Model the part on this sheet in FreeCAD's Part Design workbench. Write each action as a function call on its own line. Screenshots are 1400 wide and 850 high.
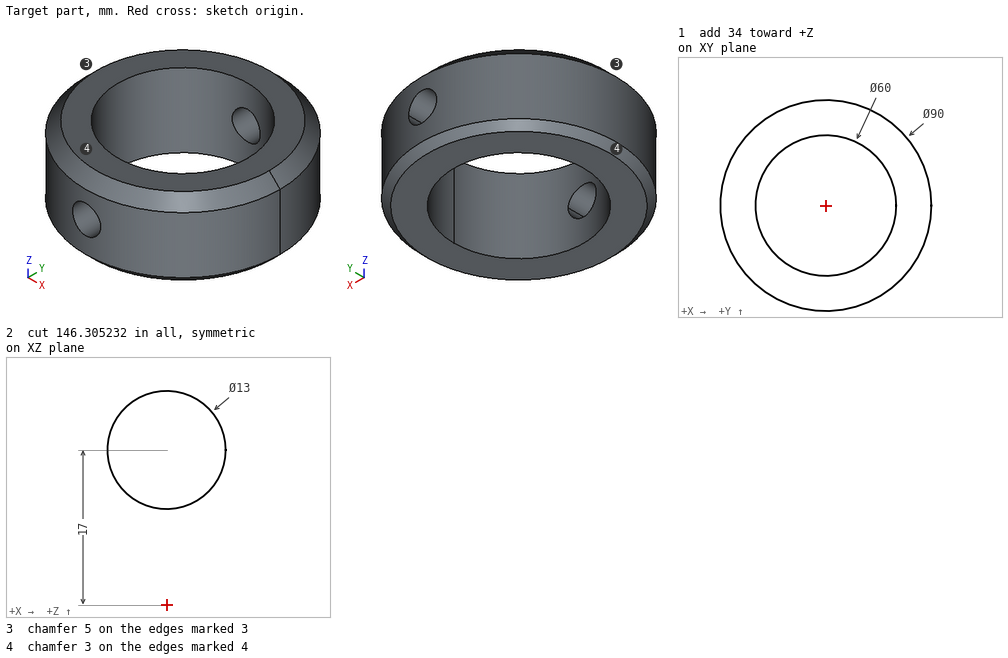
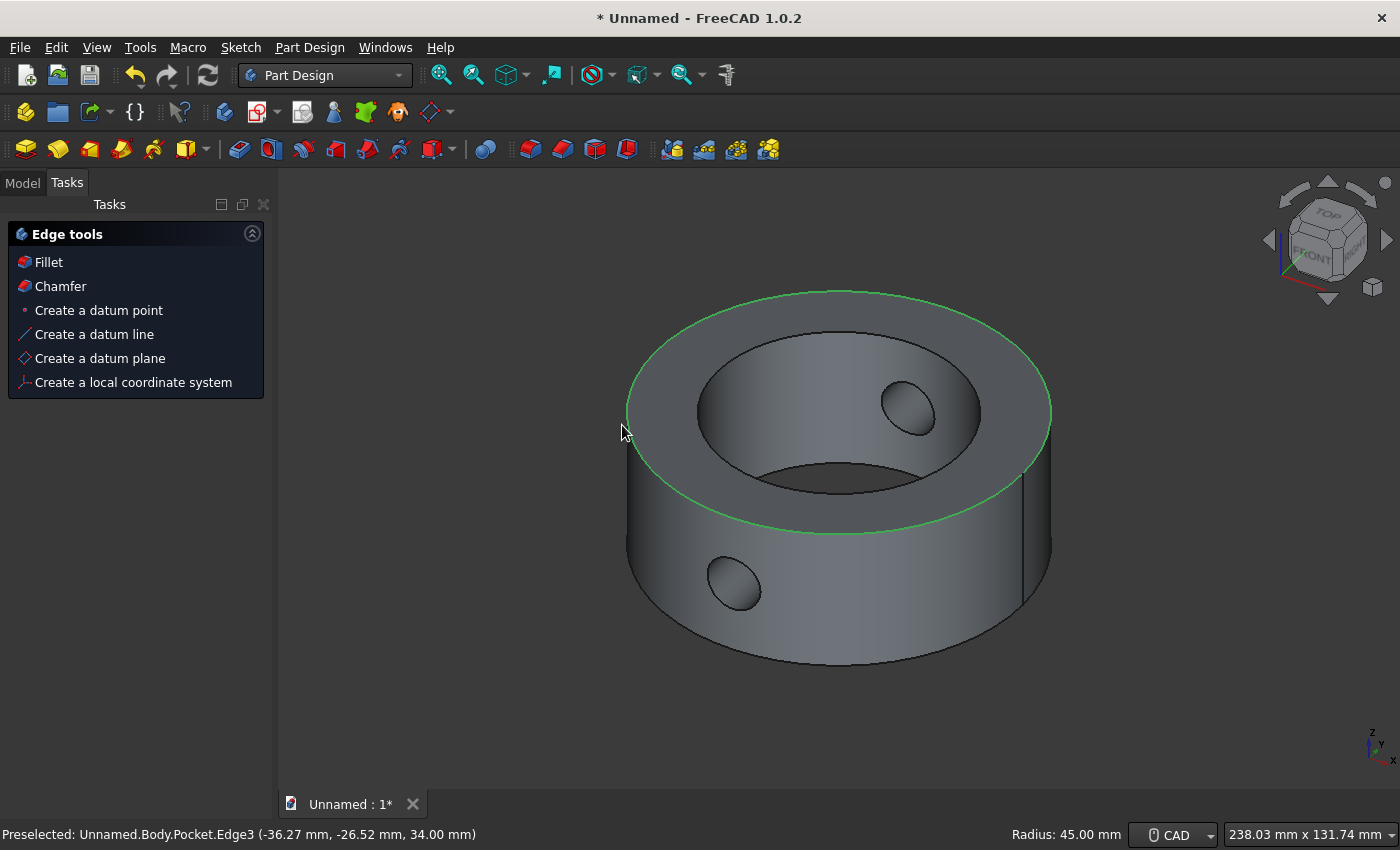
click(564, 150)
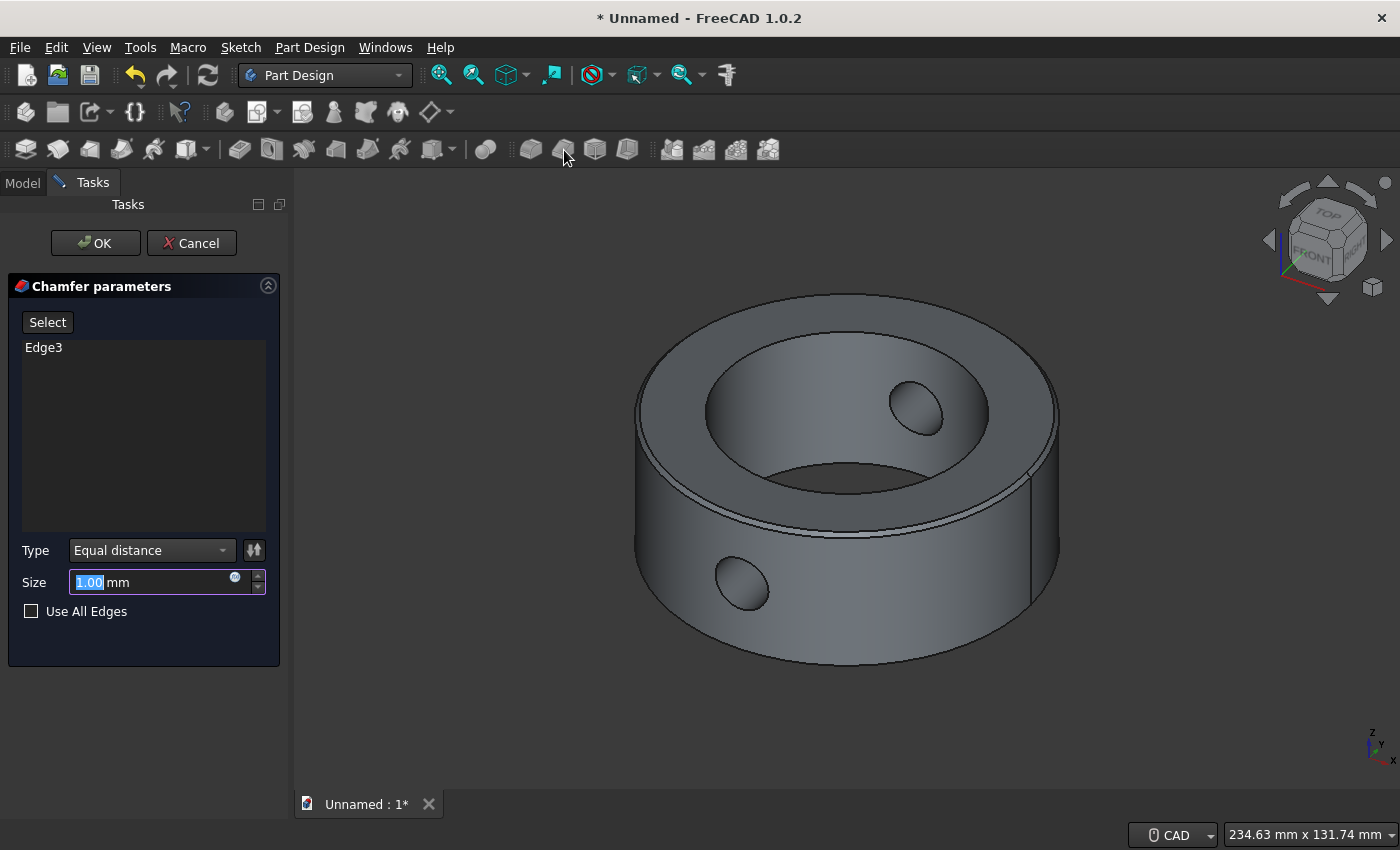
text(5)
key(Tab)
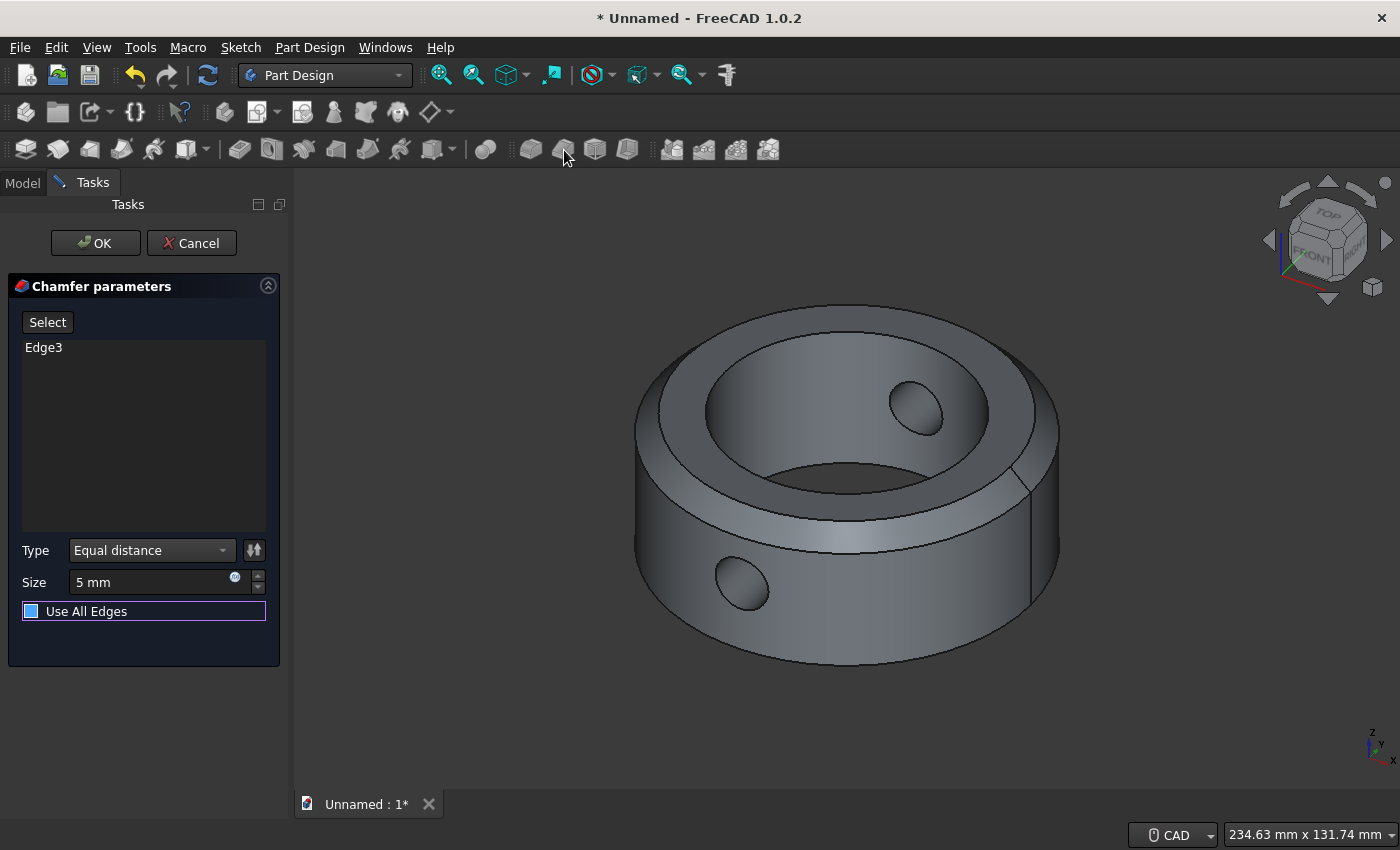
click(96, 243)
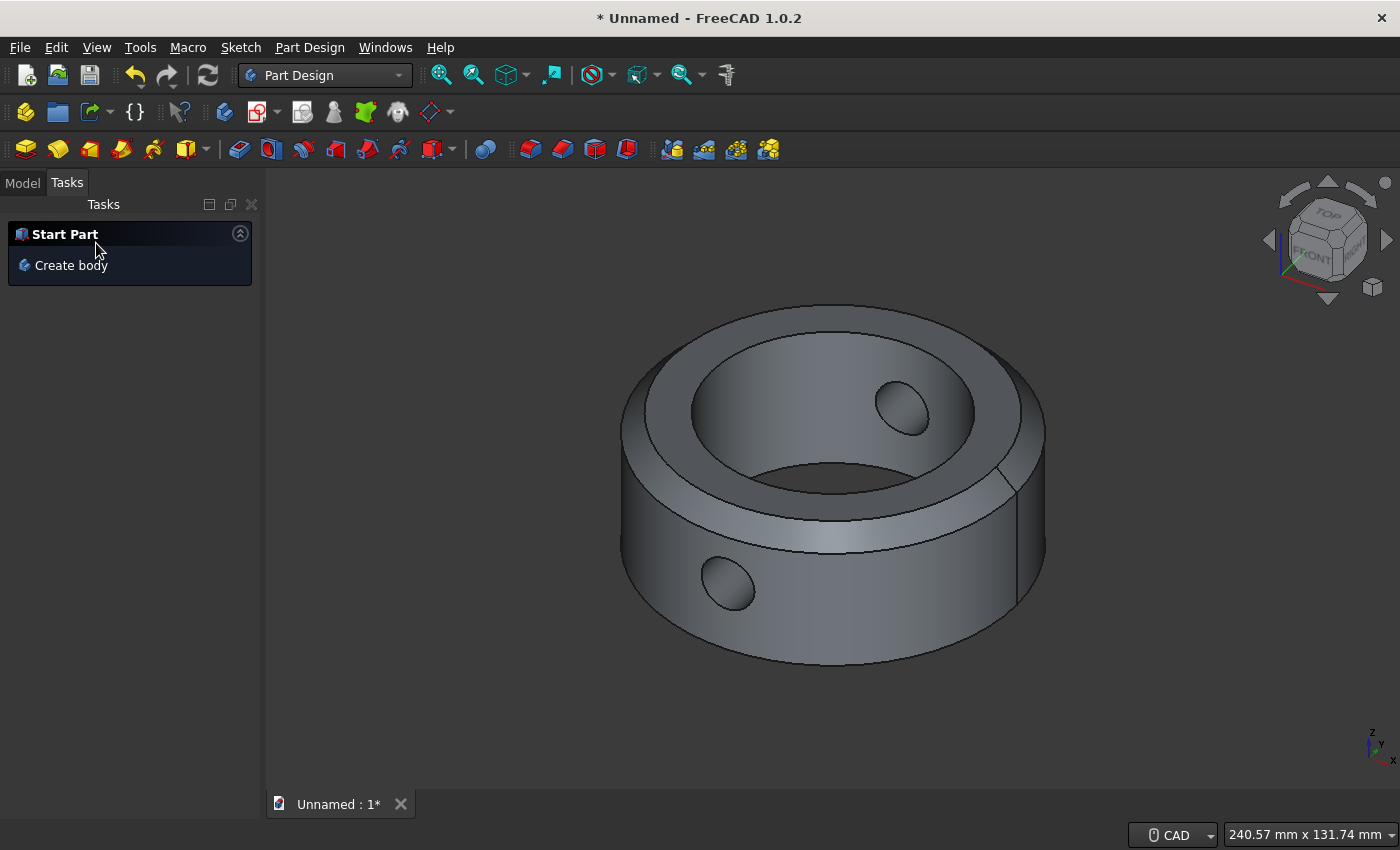
key(0)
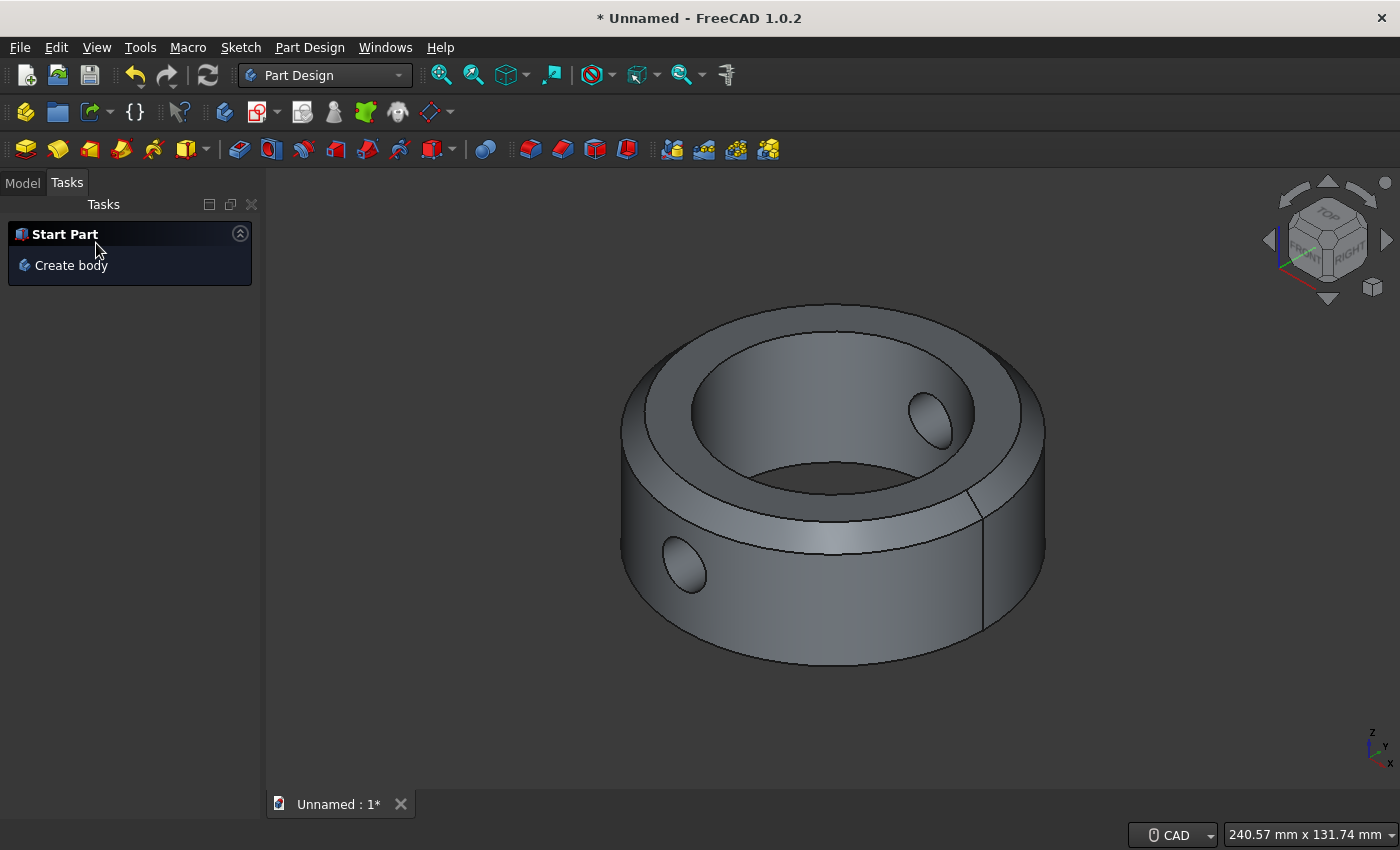
key(2)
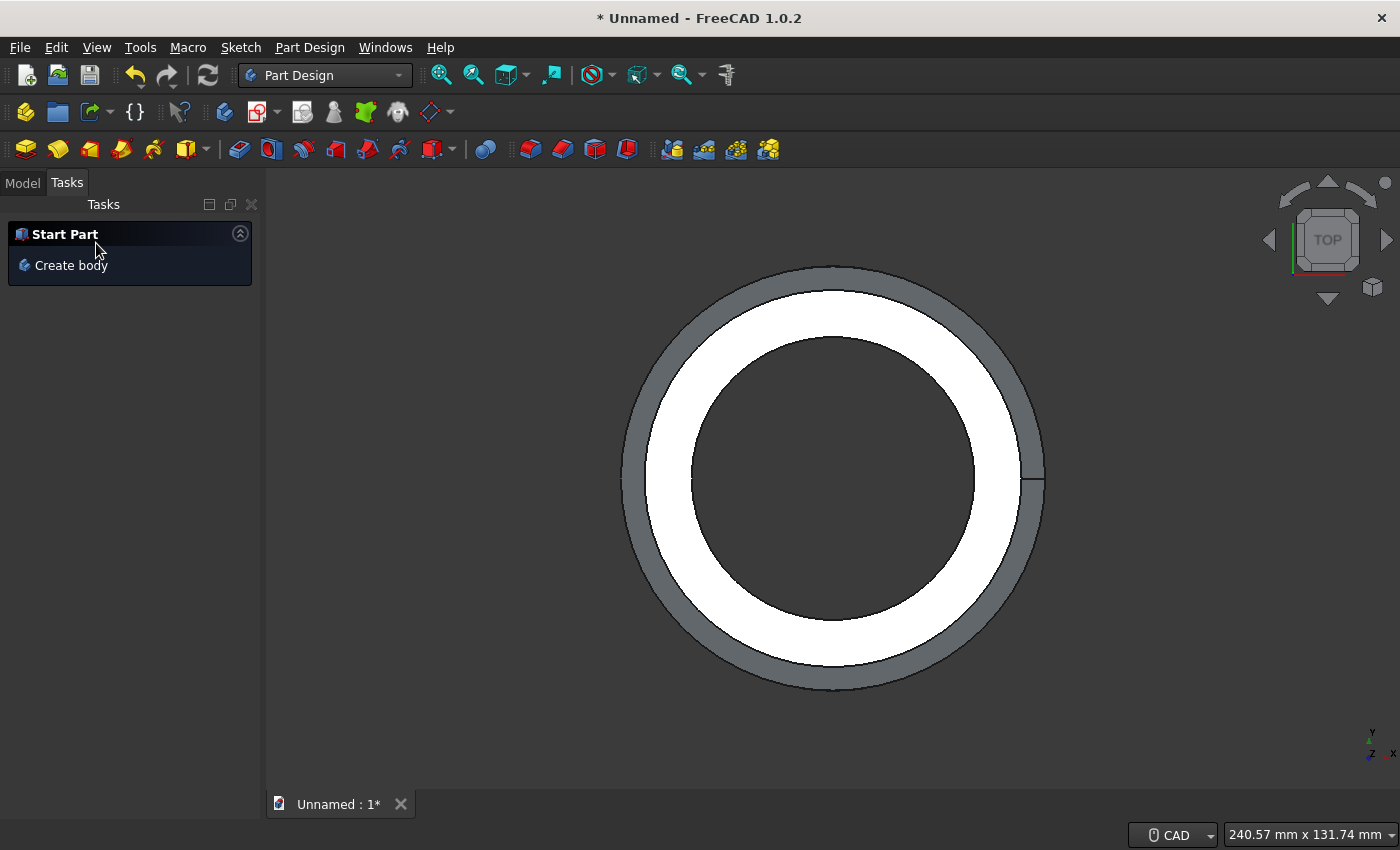
key(1)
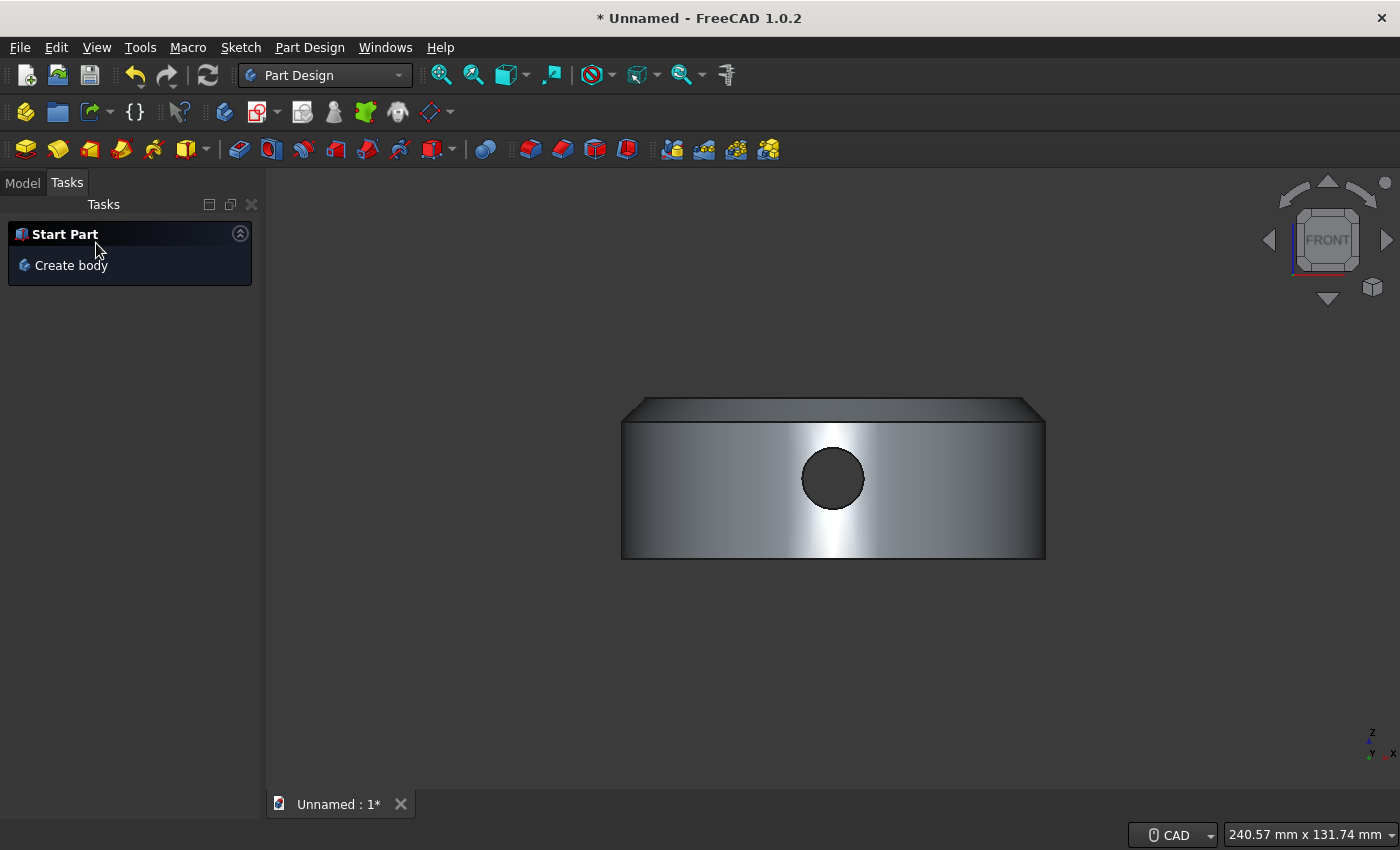
key(v)
key(f)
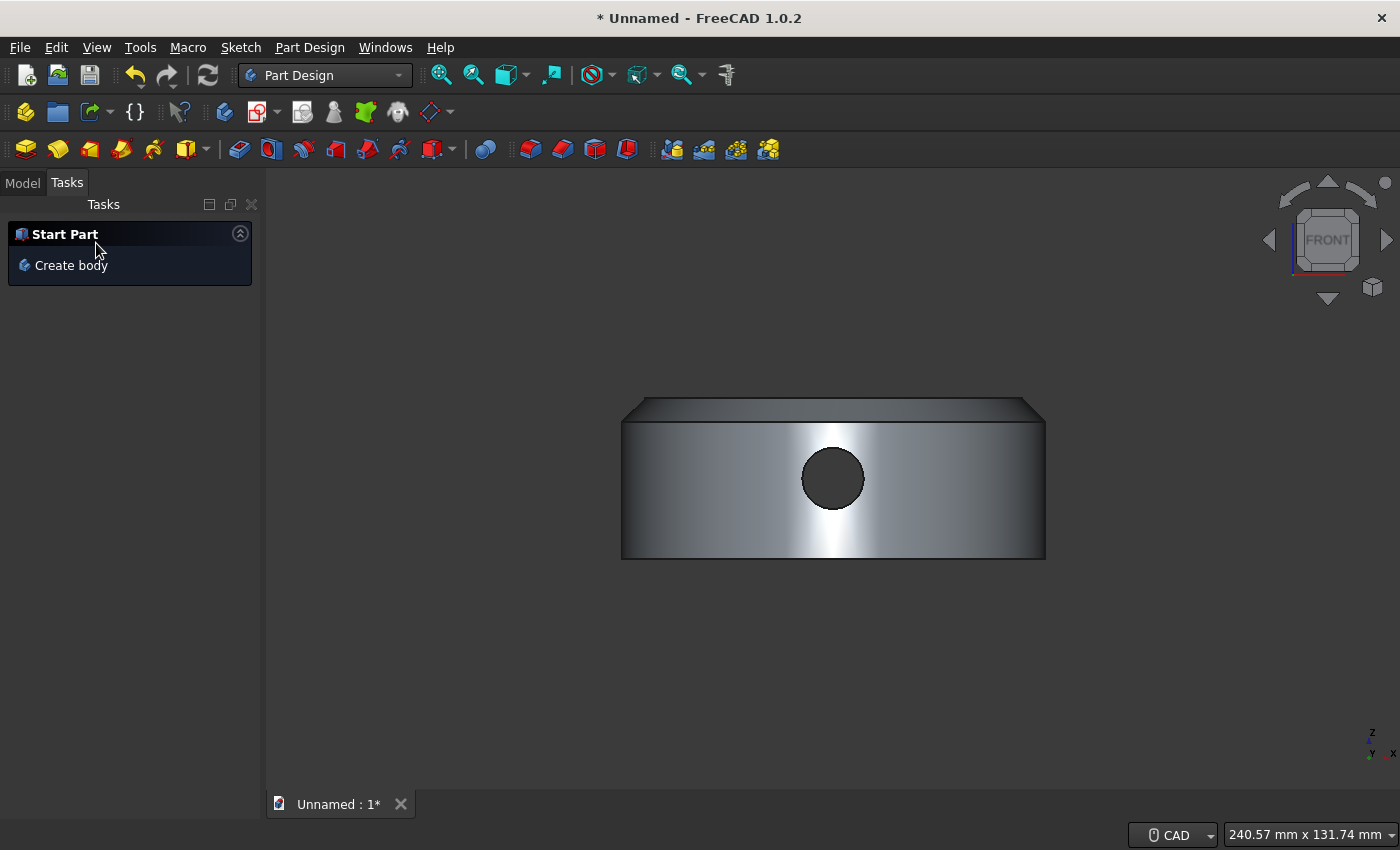
click(661, 558)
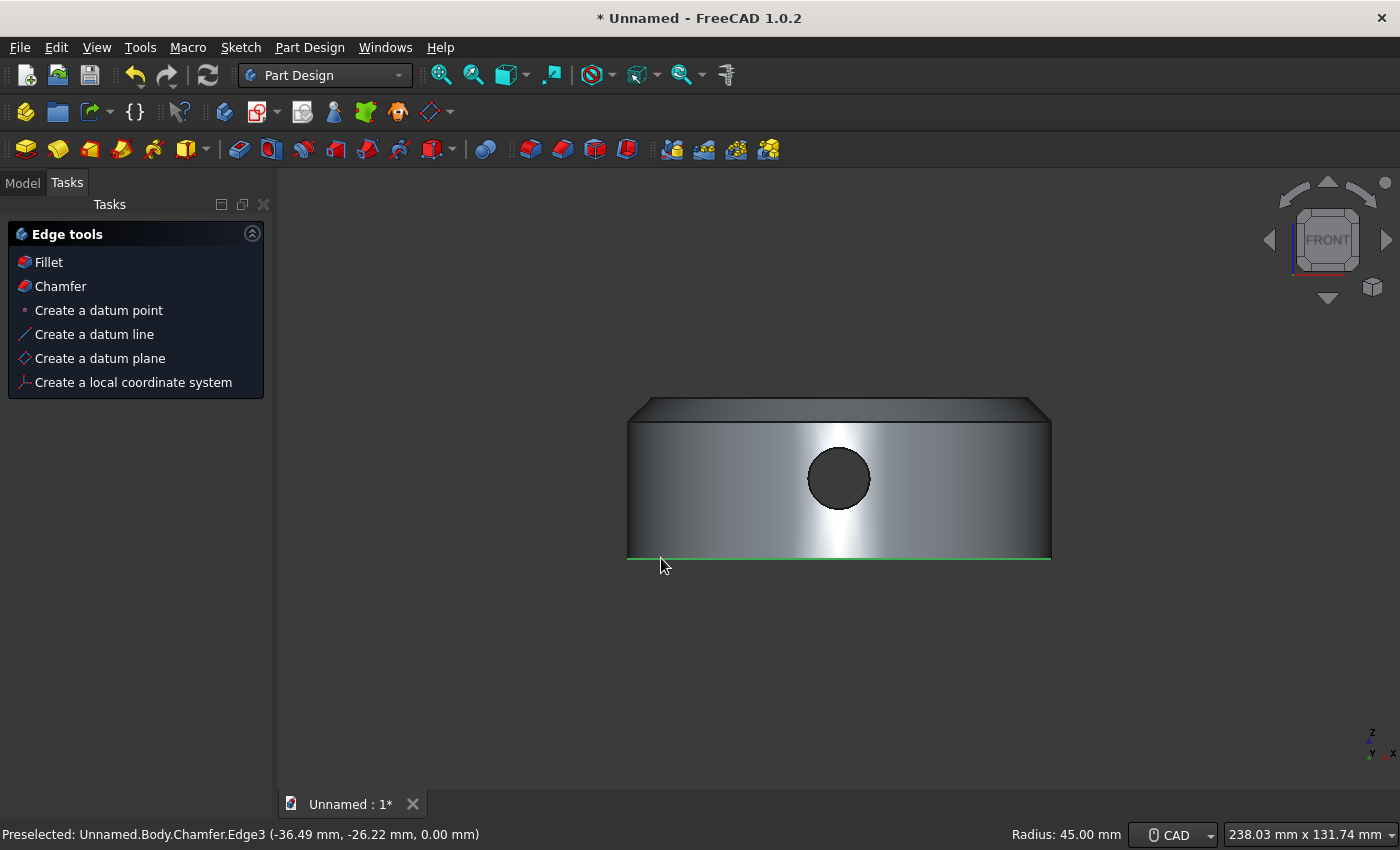
click(564, 150)